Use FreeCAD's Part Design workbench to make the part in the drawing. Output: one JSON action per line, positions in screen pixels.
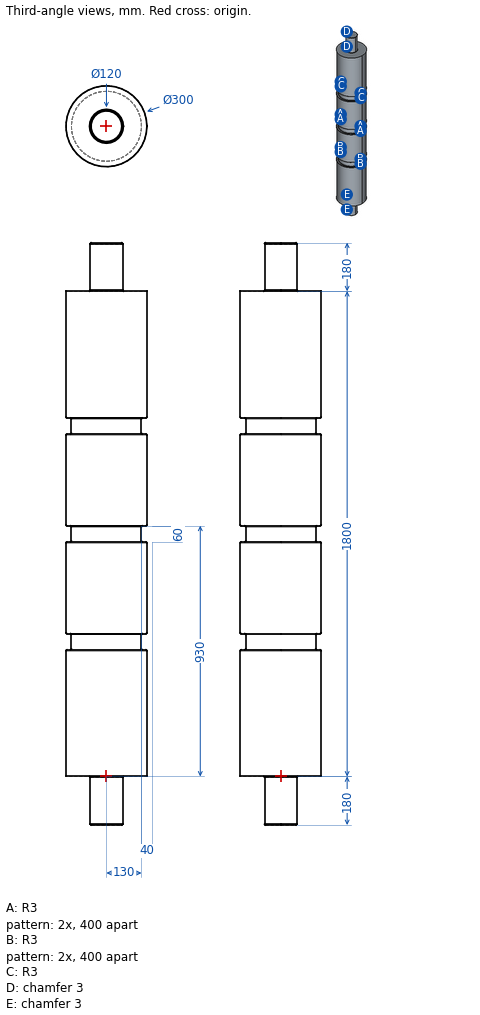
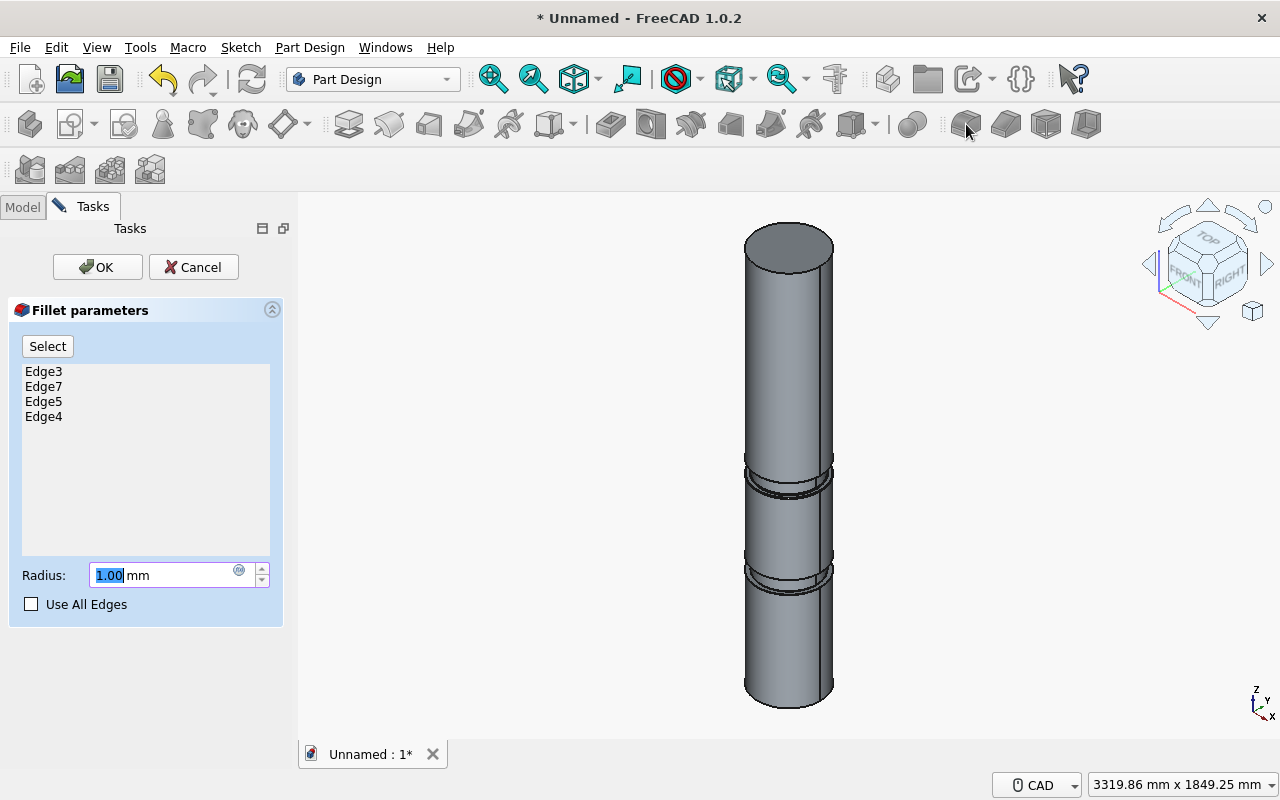
{"action": "type", "text": "3"}
{"action": "key", "text": "Tab"}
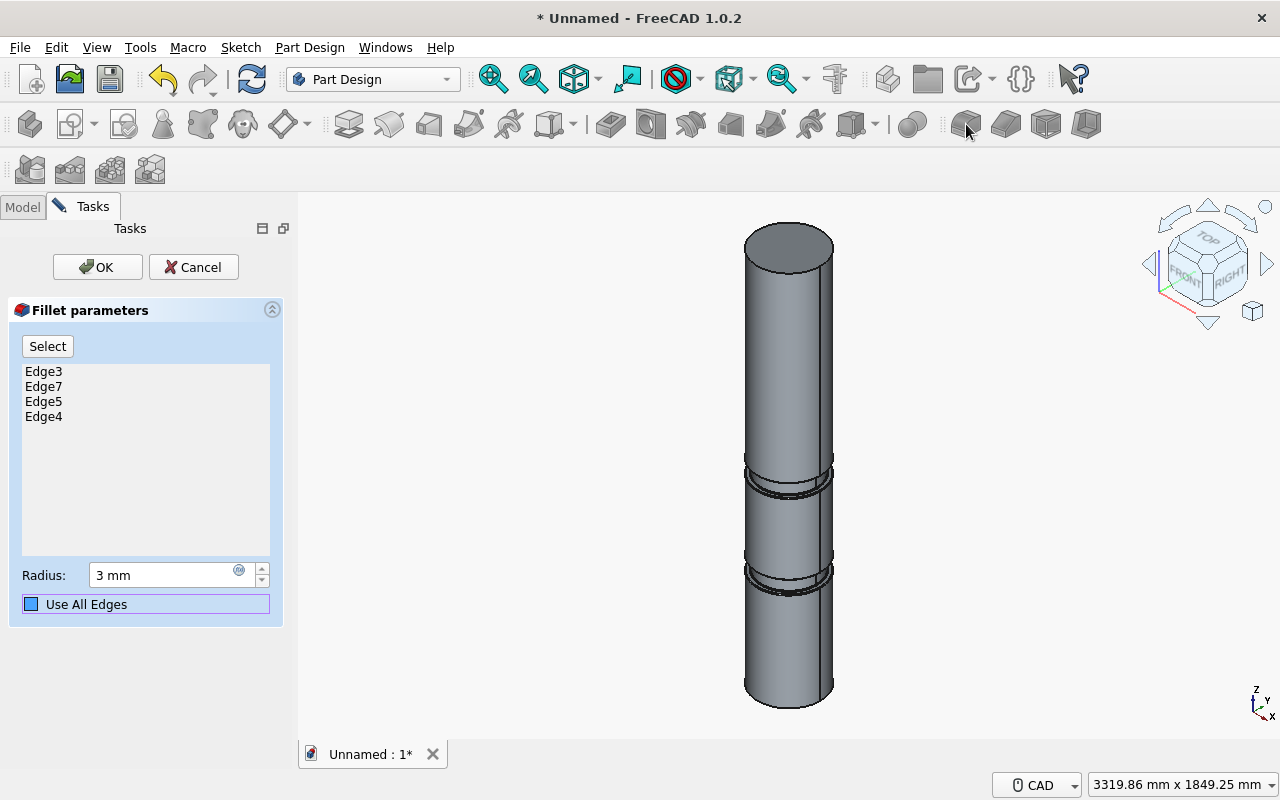
{"action": "left_click", "coordinate": [98, 267]}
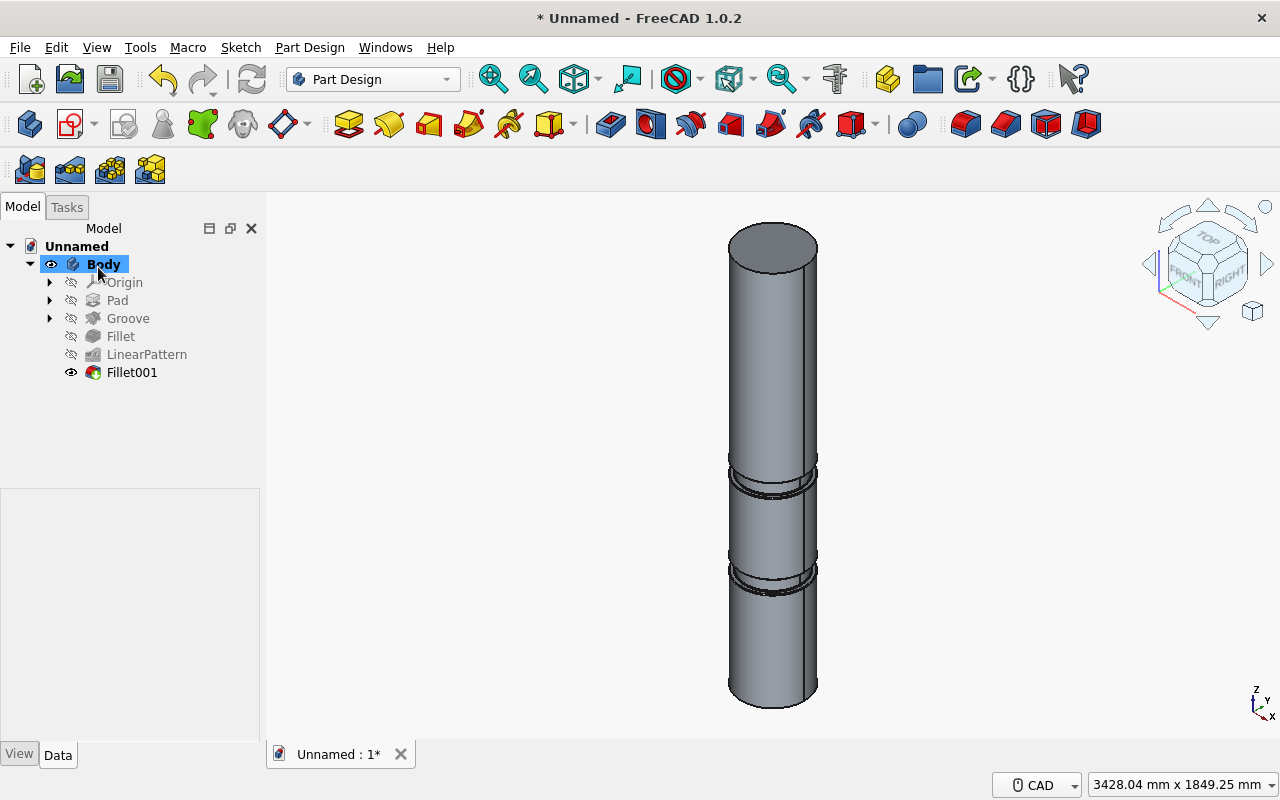
{"action": "left_click", "coordinate": [116, 318]}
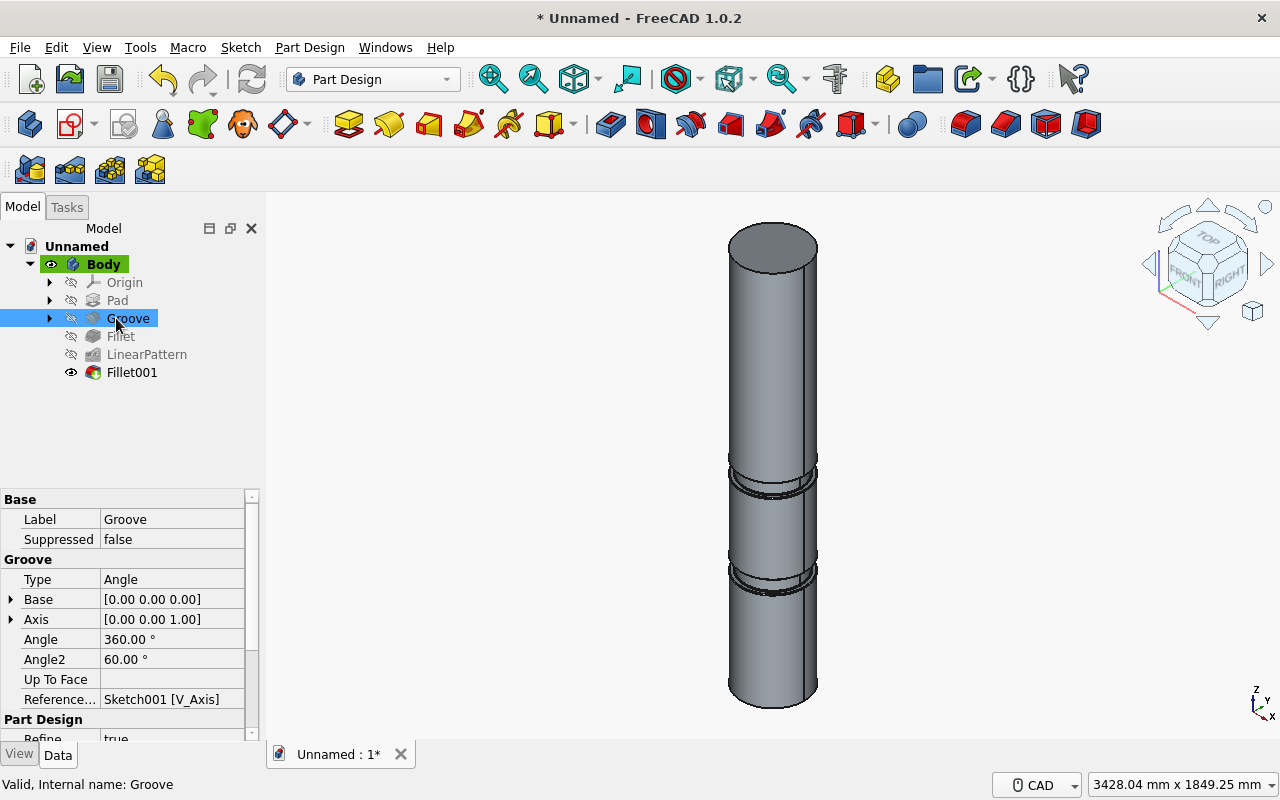
{"action": "left_click", "coordinate": [70, 170]}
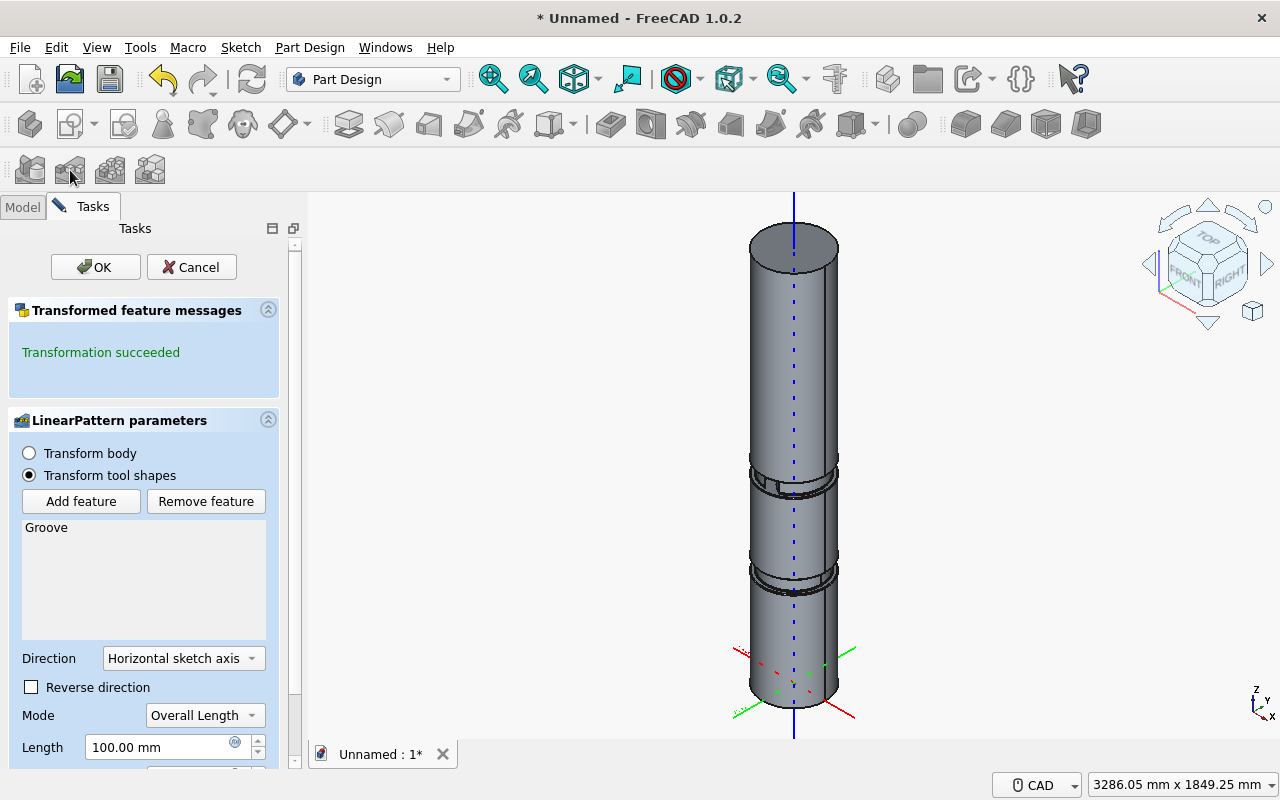
{"action": "left_click", "coordinate": [184, 658]}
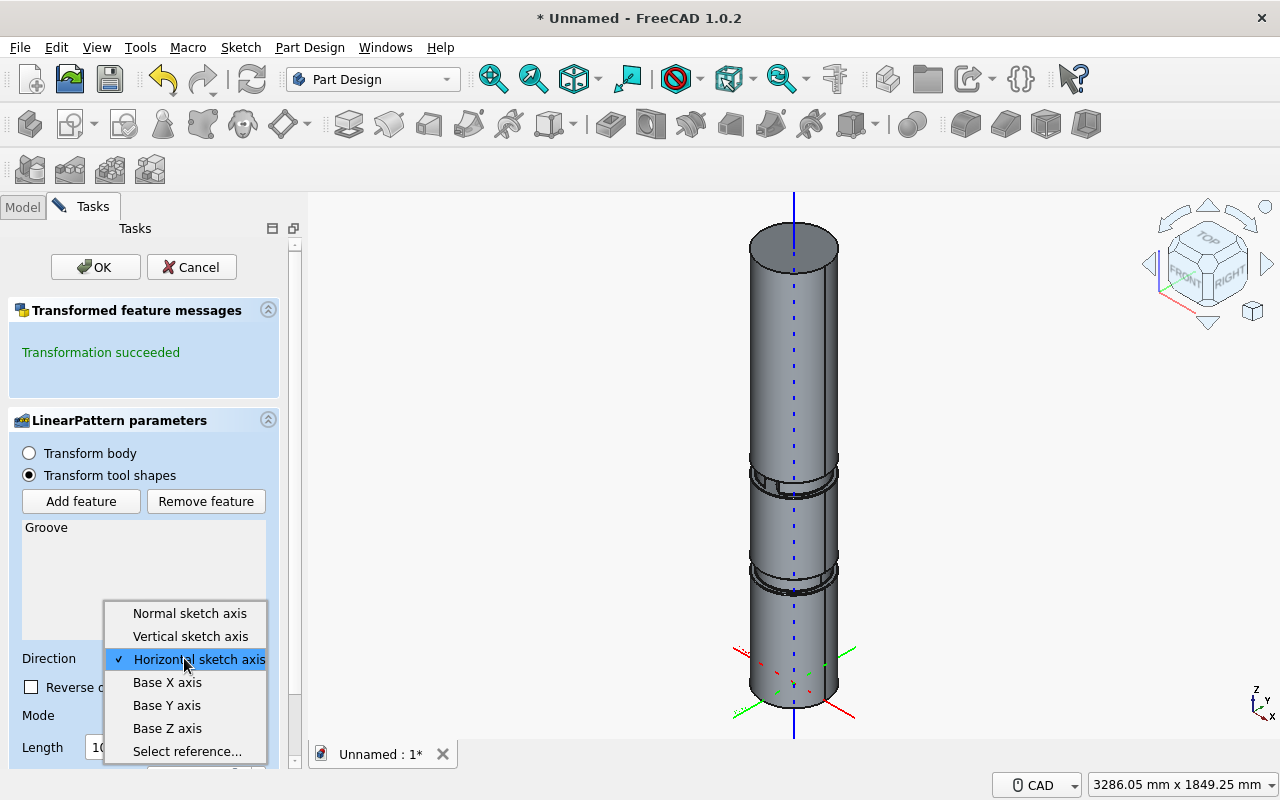
{"action": "left_click", "coordinate": [184, 728]}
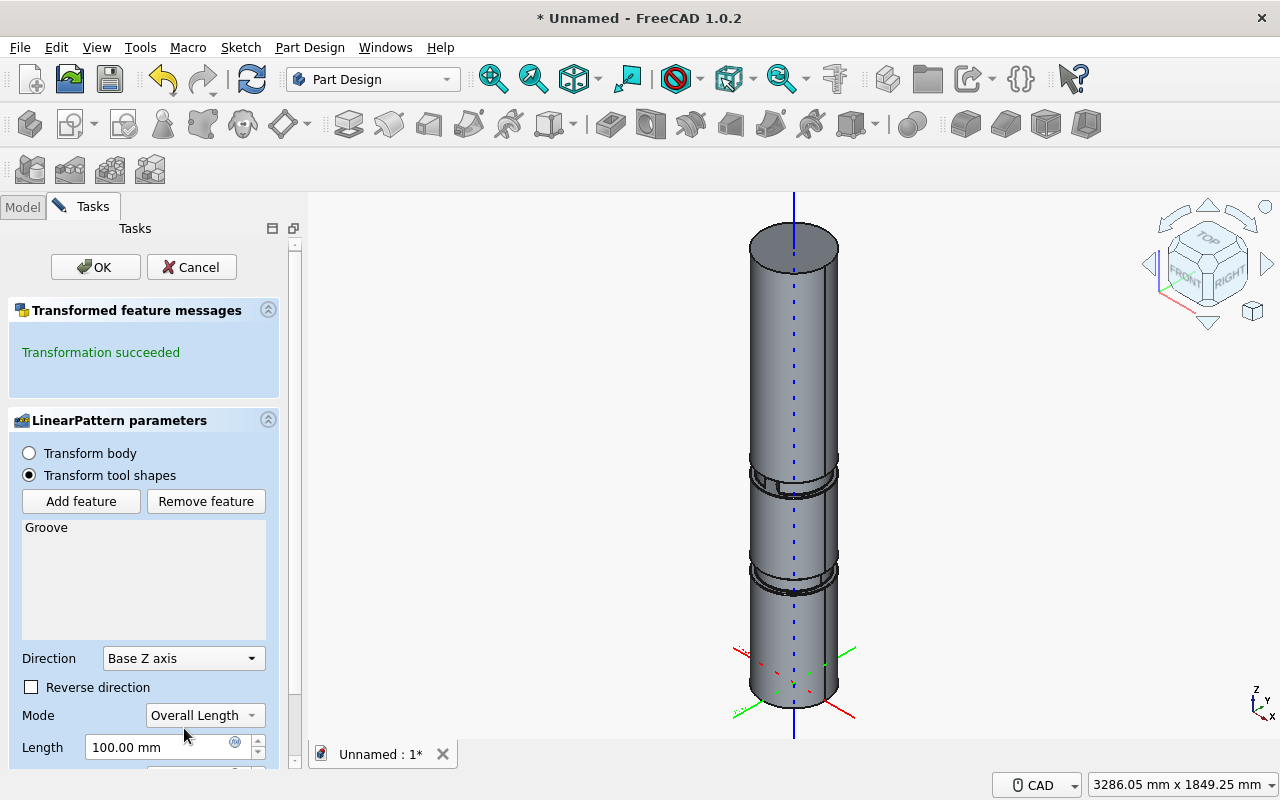
{"action": "left_click", "coordinate": [206, 716]}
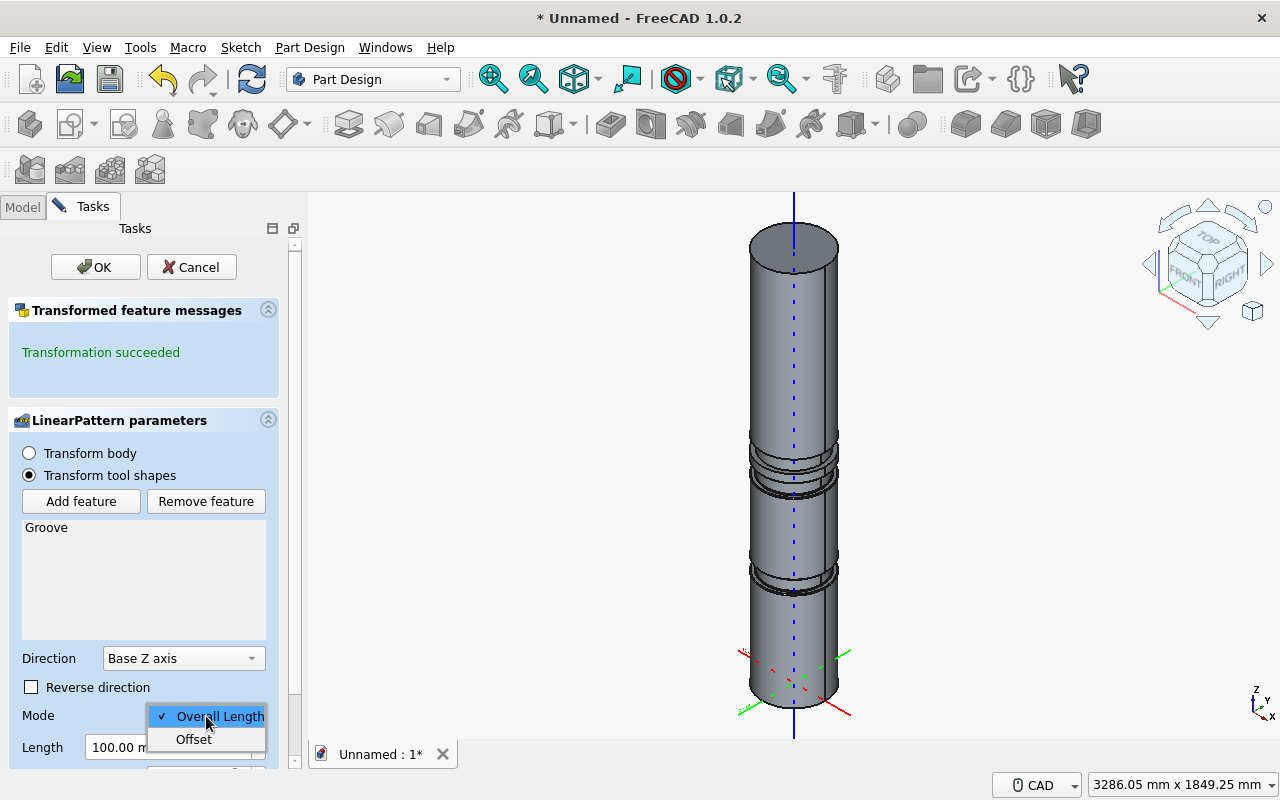
{"action": "left_click", "coordinate": [206, 740]}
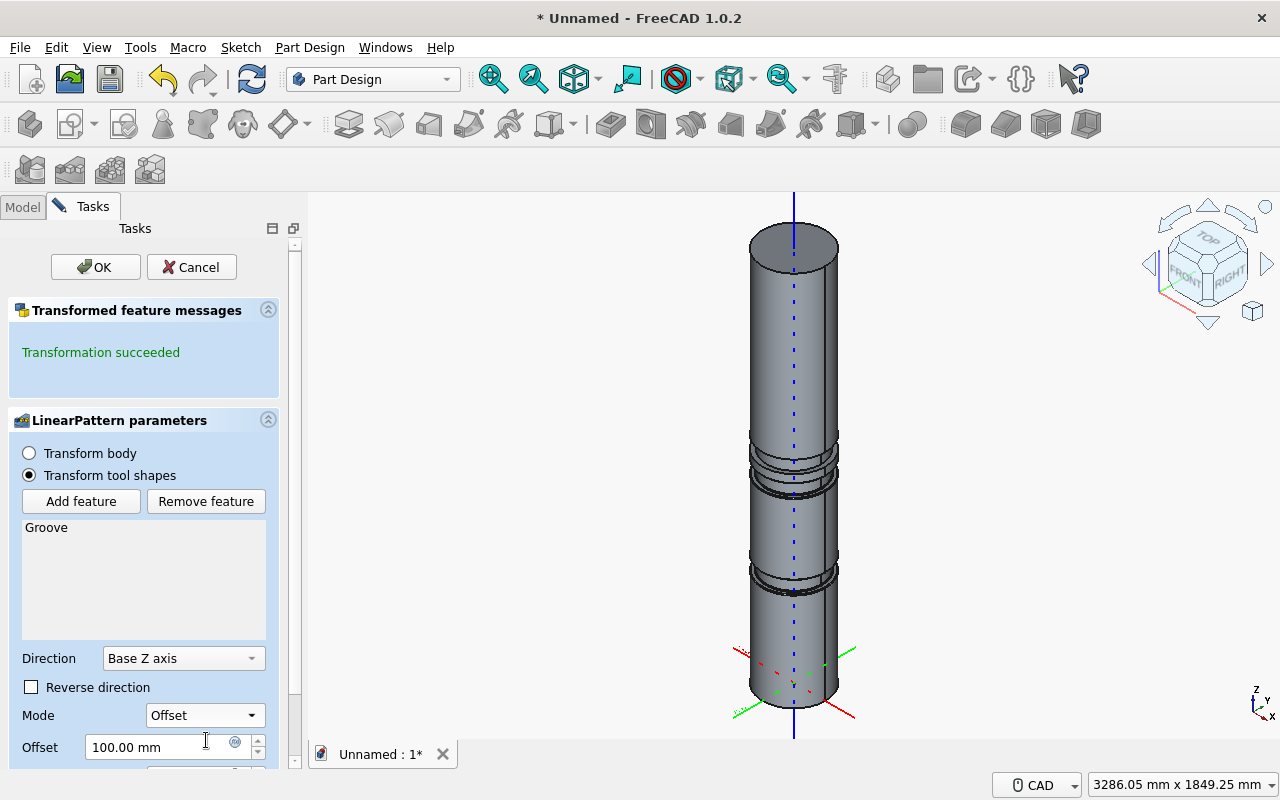
{"action": "triple_click", "coordinate": [168, 747]}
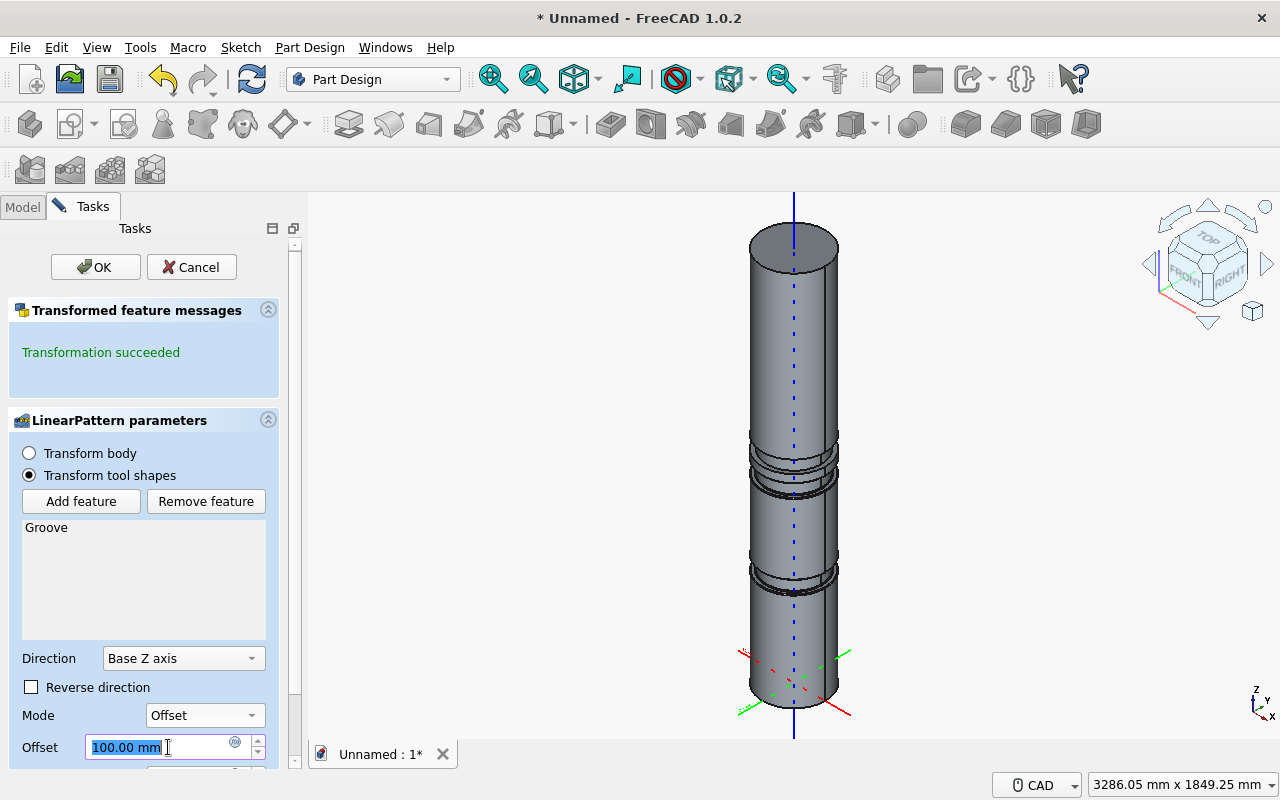
{"action": "type", "text": "400"}
{"action": "key", "text": "Tab"}